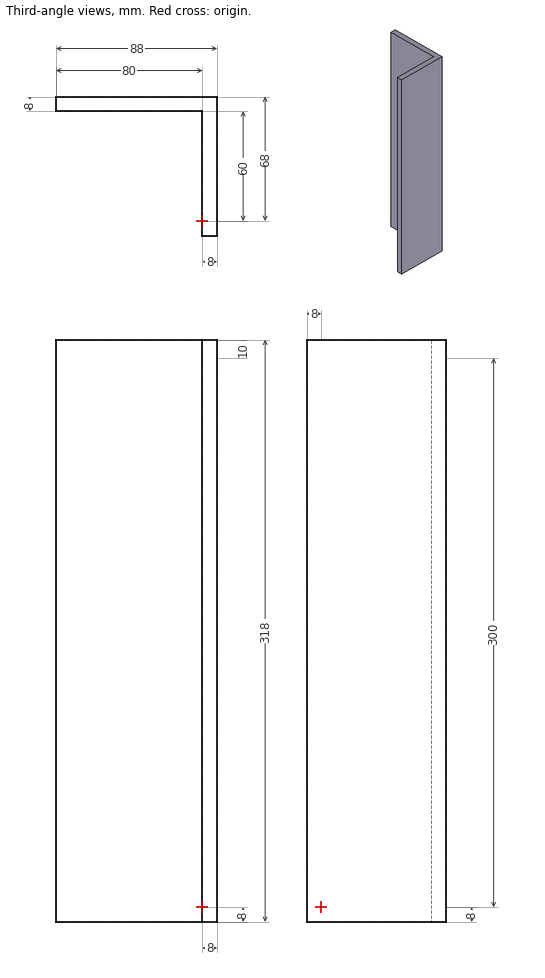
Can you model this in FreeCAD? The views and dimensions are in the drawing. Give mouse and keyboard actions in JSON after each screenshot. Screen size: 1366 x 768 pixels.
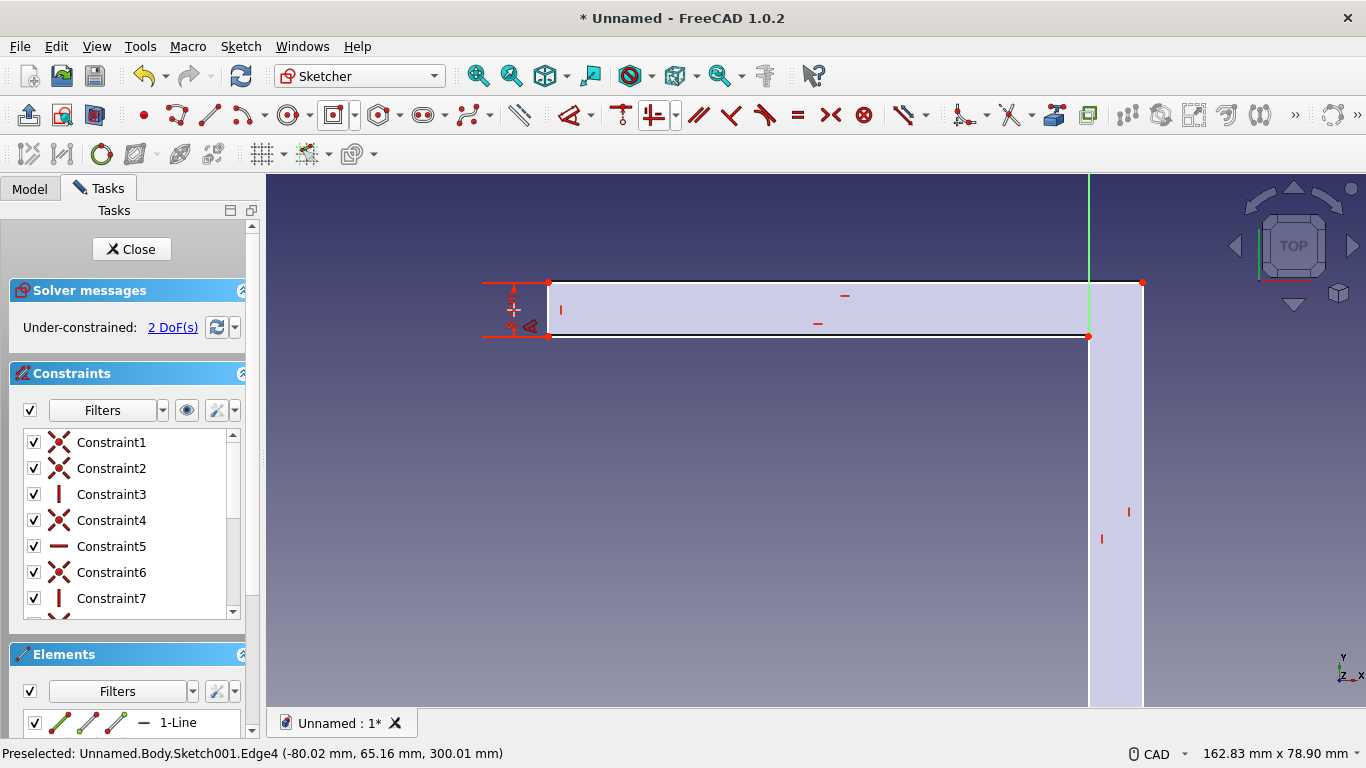
{"action": "left_click", "coordinate": [1143, 603]}
{"action": "left_click", "coordinate": [1177, 481]}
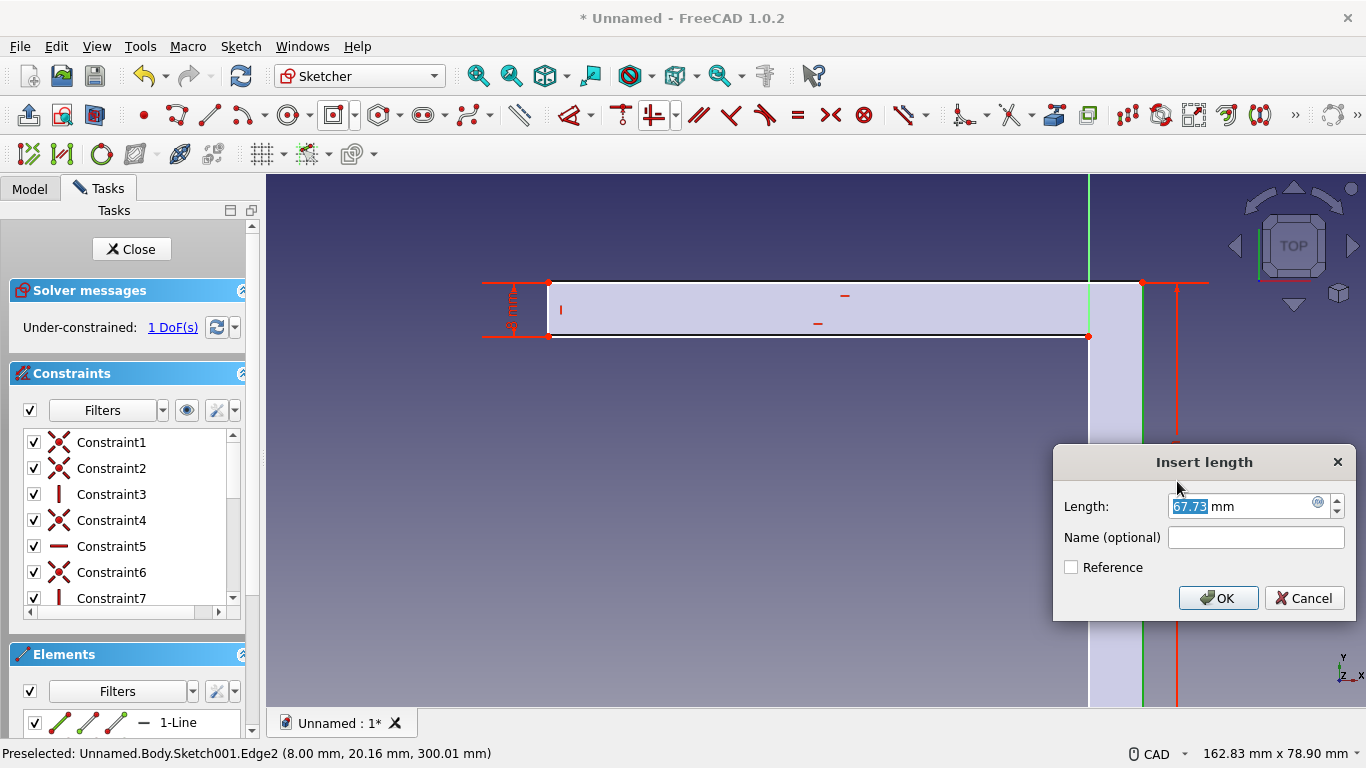
{"action": "type", "text": "68"}
{"action": "key", "text": "Return"}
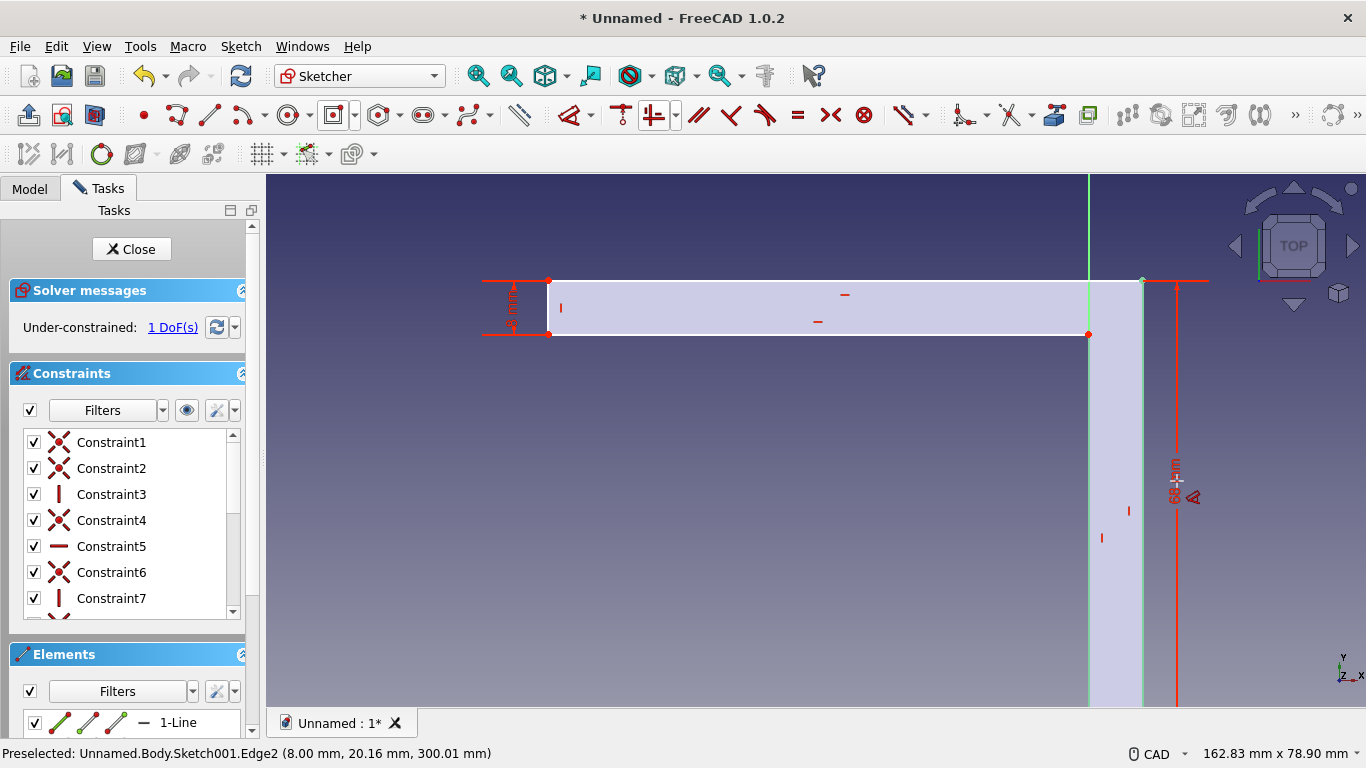
{"action": "left_click", "coordinate": [965, 281]}
{"action": "left_click", "coordinate": [846, 247]}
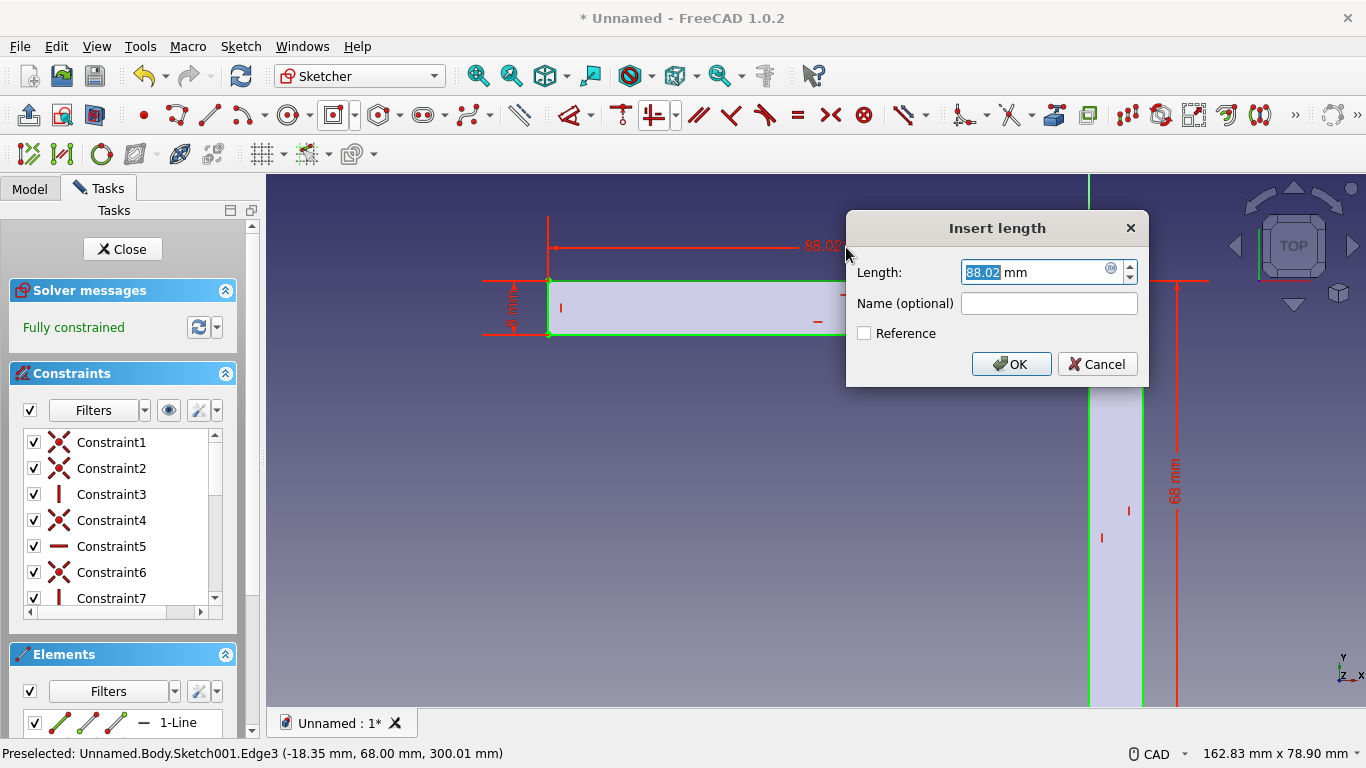
{"action": "type", "text": "88"}
{"action": "key", "text": "Return"}
{"action": "key", "text": "Escape"}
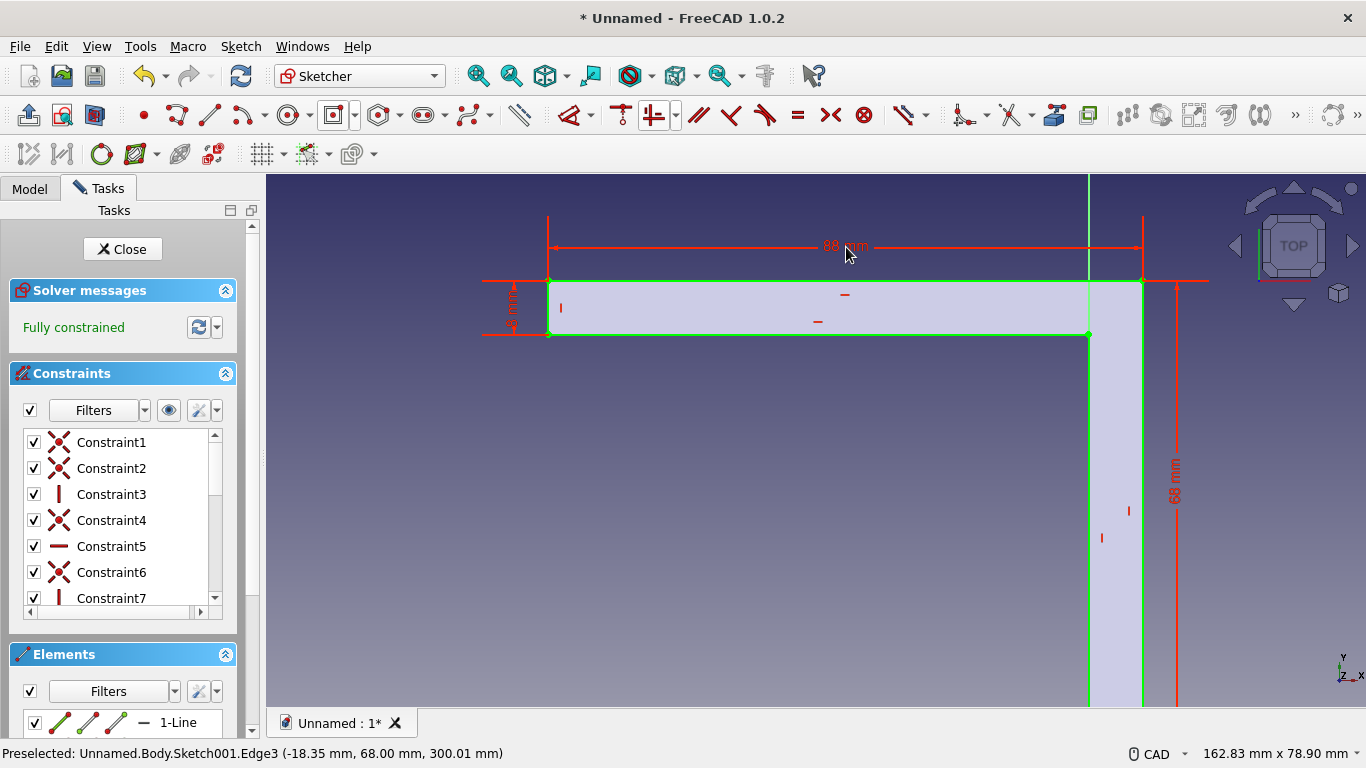
{"action": "left_click", "coordinate": [123, 249]}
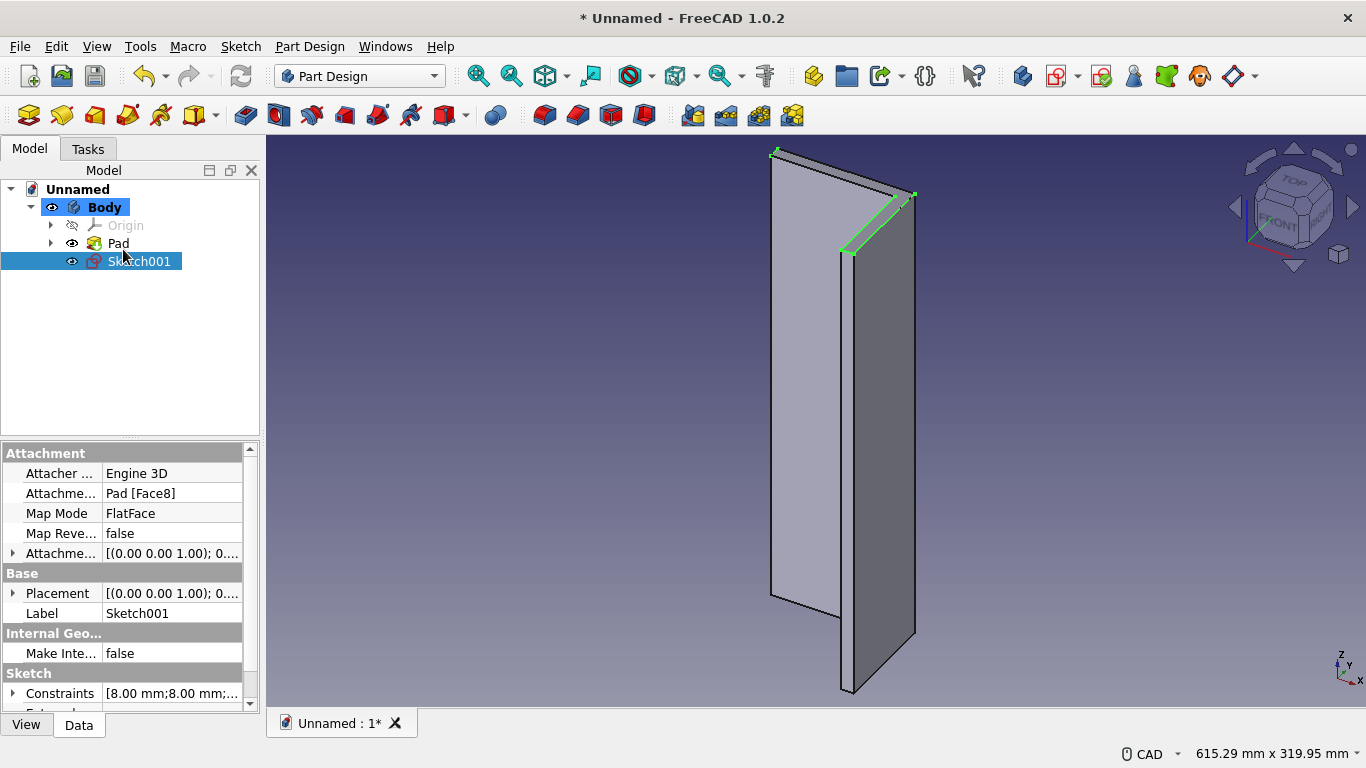
{"action": "left_click", "coordinate": [29, 116]}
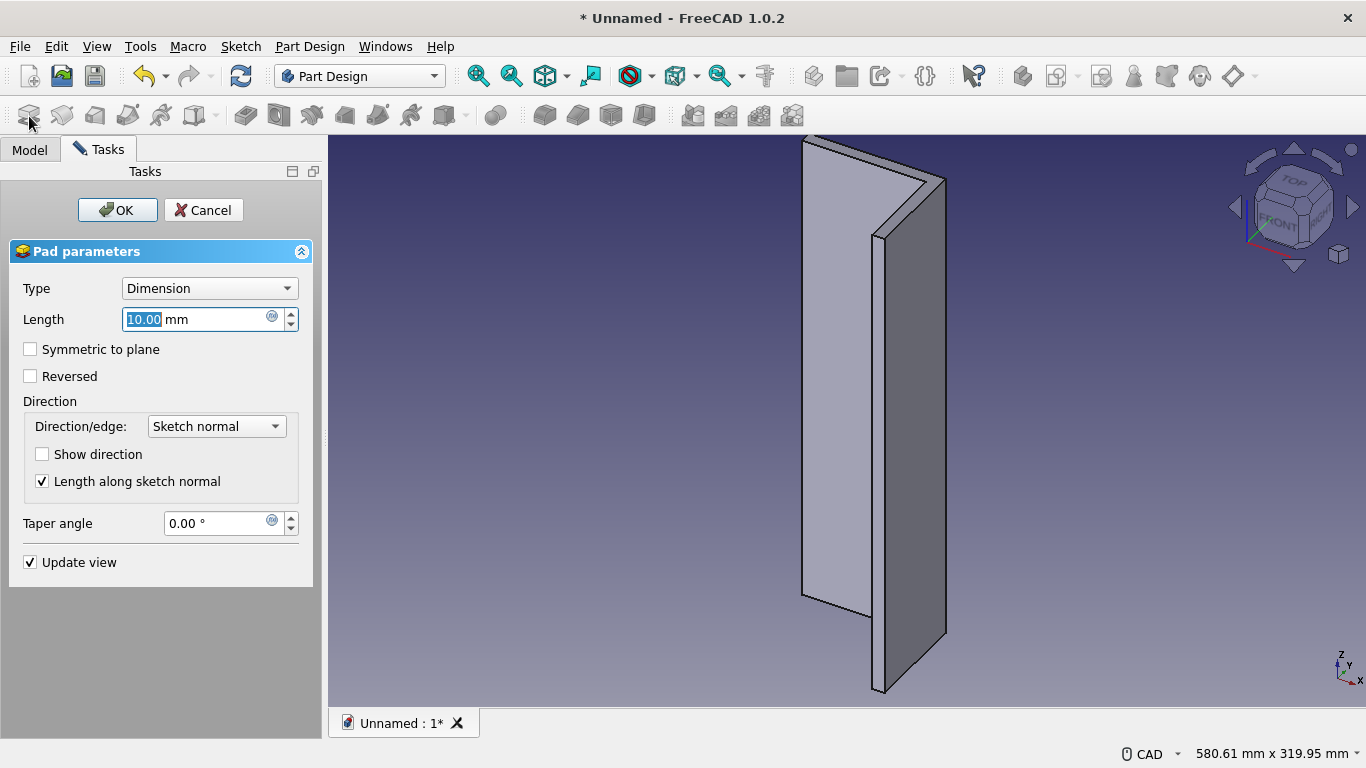
{"action": "type", "text": "10"}
{"action": "key", "text": "Tab"}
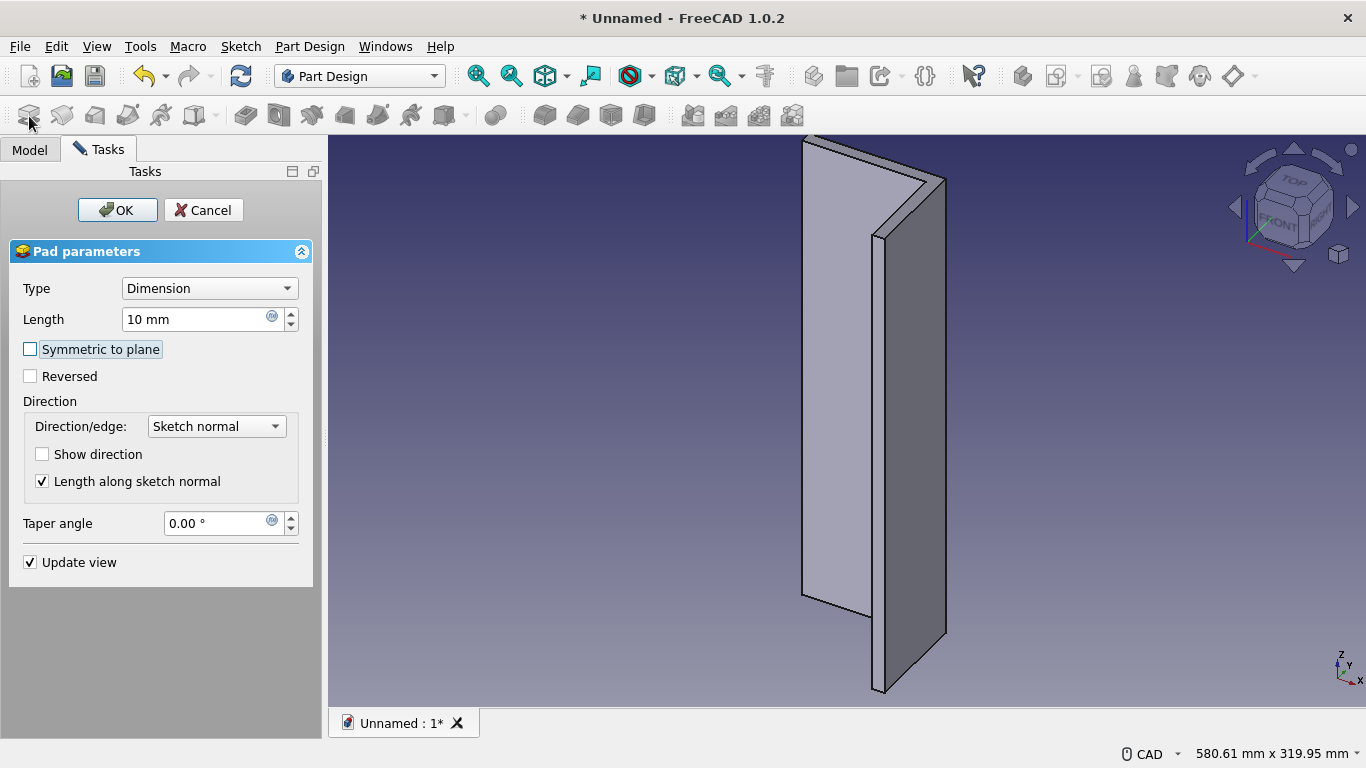
{"action": "left_click", "coordinate": [118, 210]}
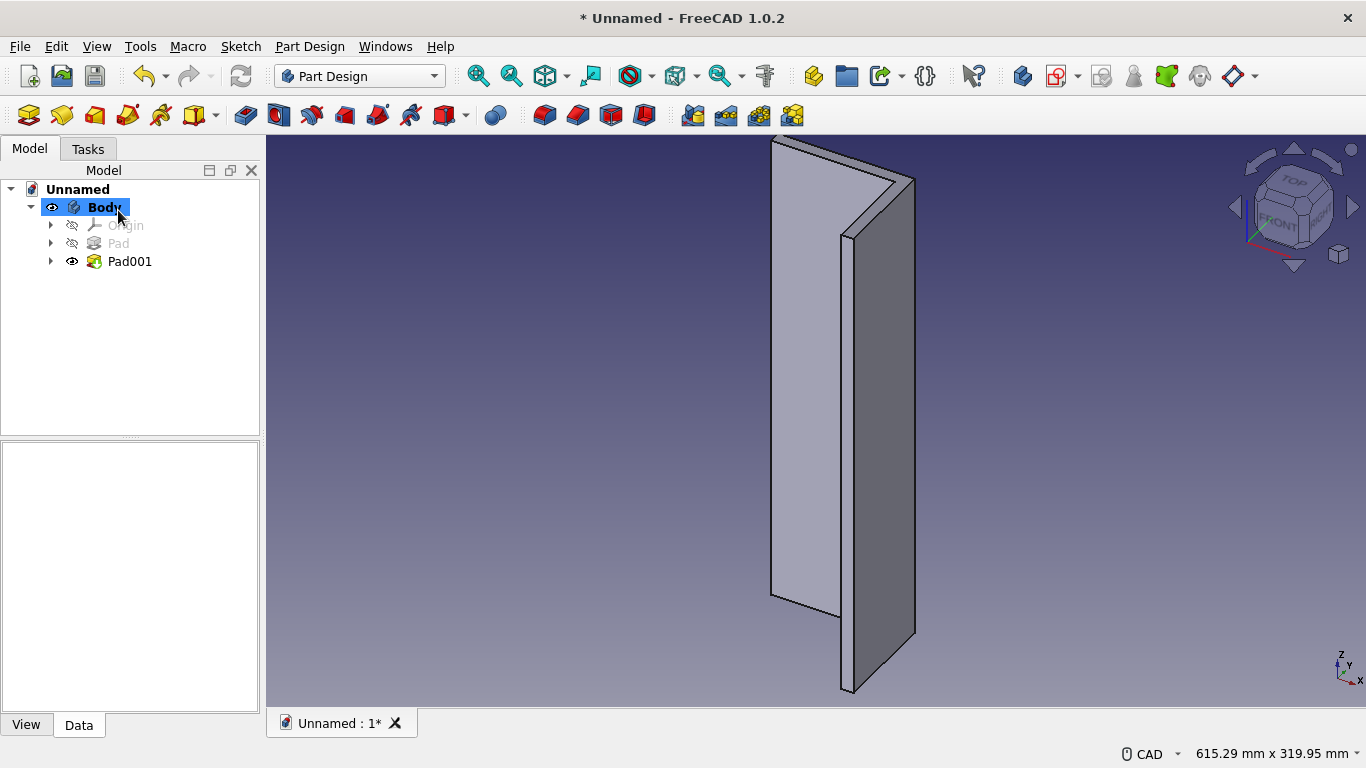
{"action": "left_click", "coordinate": [479, 76]}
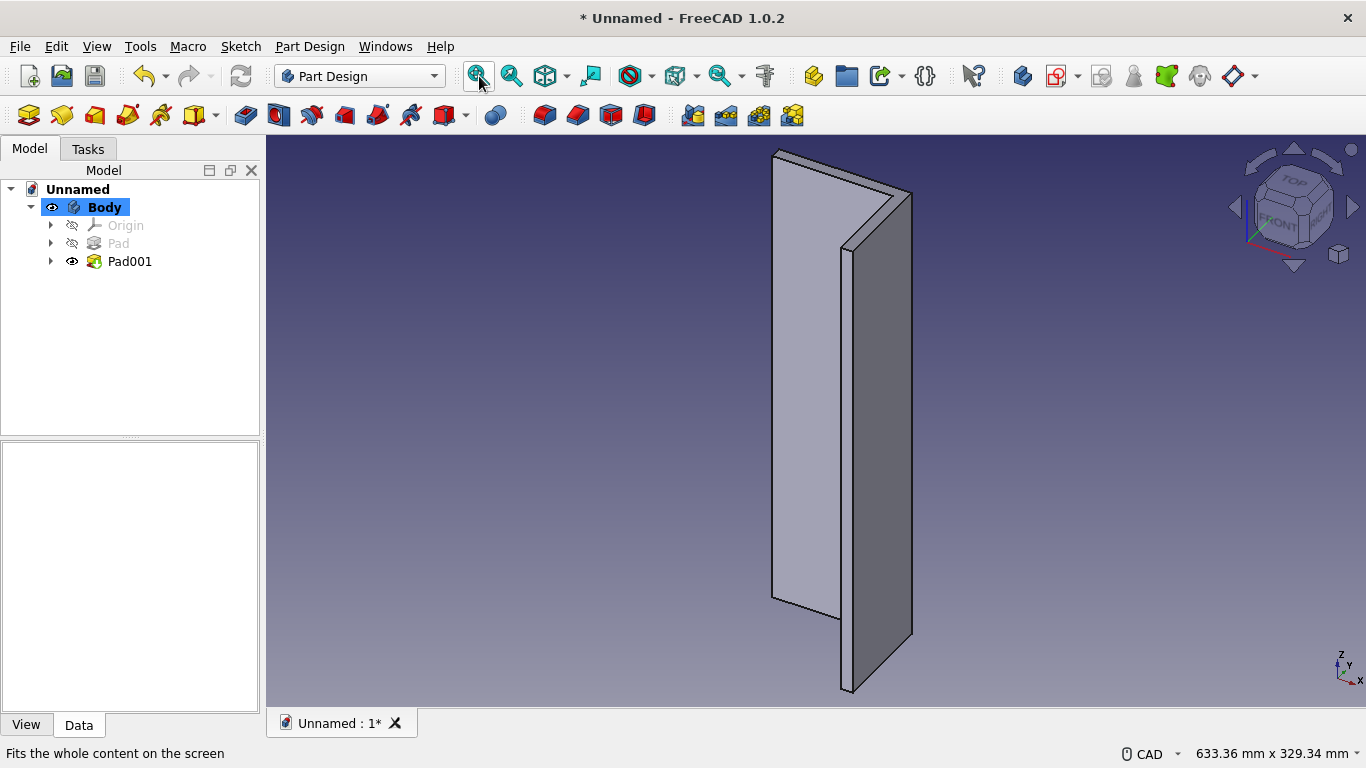
{"action": "key", "text": "5"}